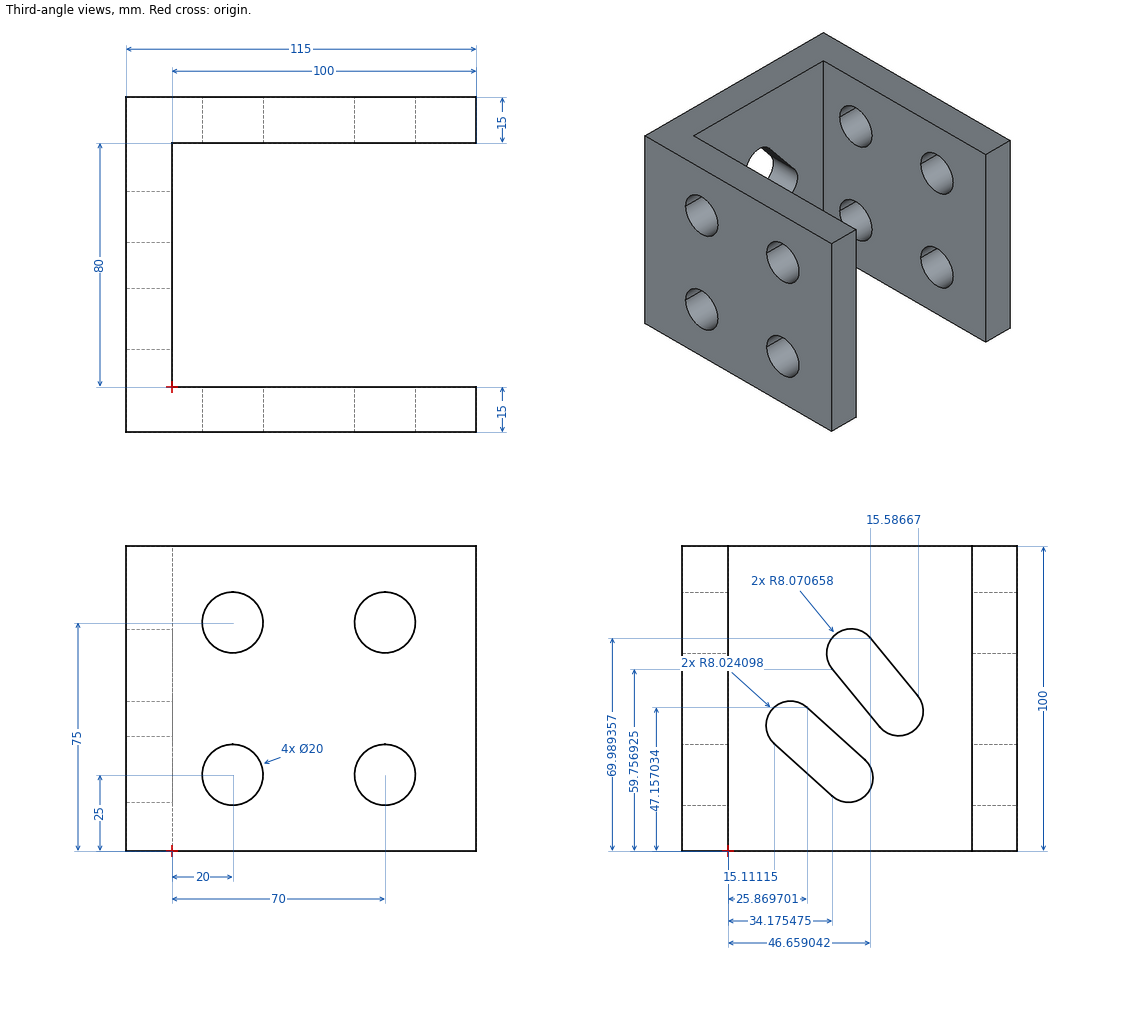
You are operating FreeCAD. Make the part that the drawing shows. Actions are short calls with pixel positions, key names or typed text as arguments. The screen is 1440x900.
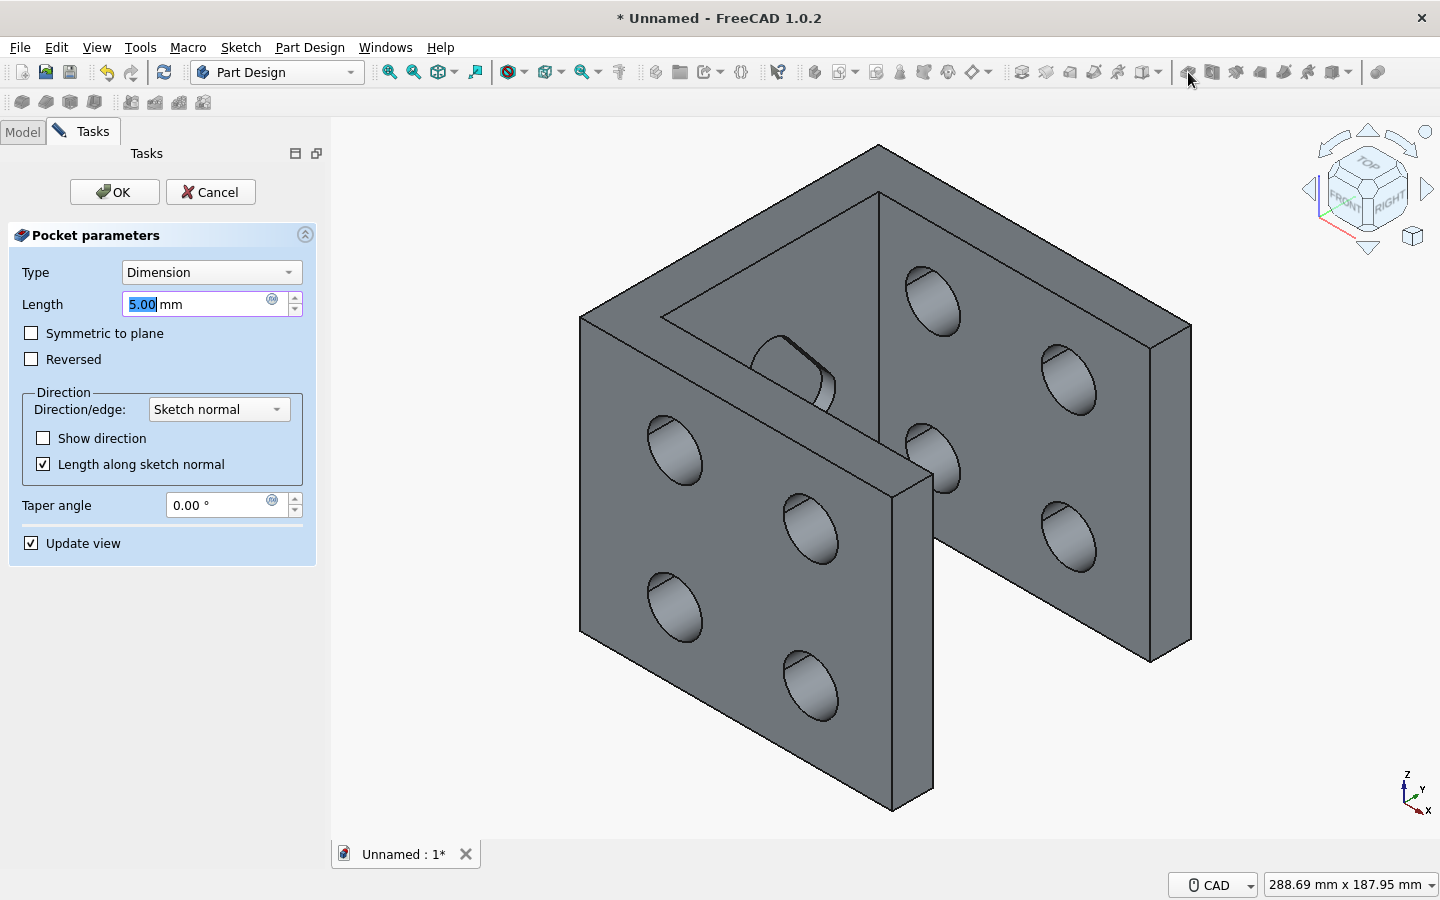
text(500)
key(Tab)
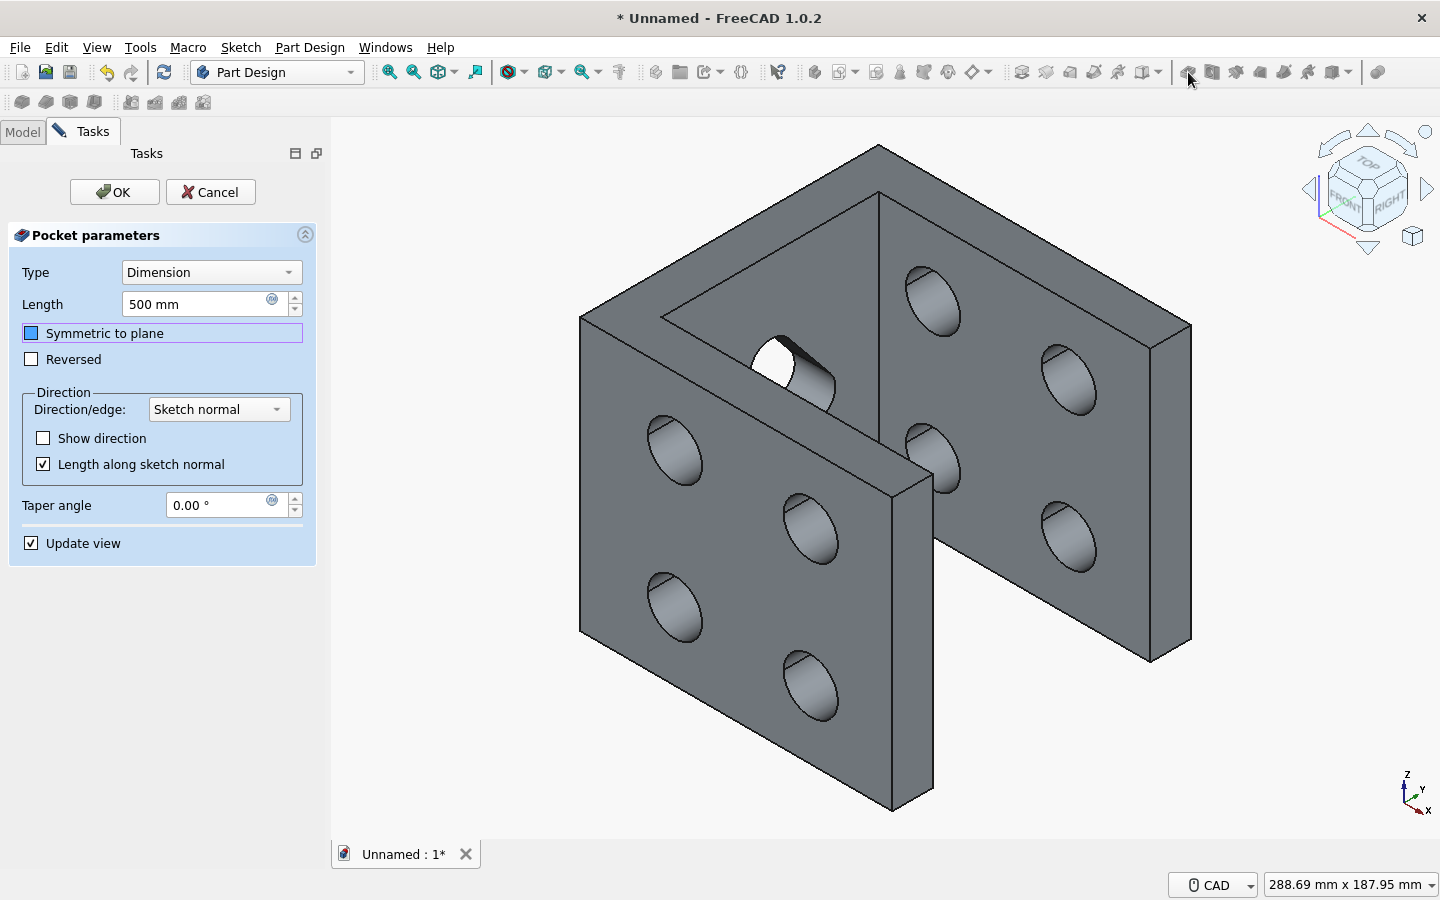
click(115, 192)